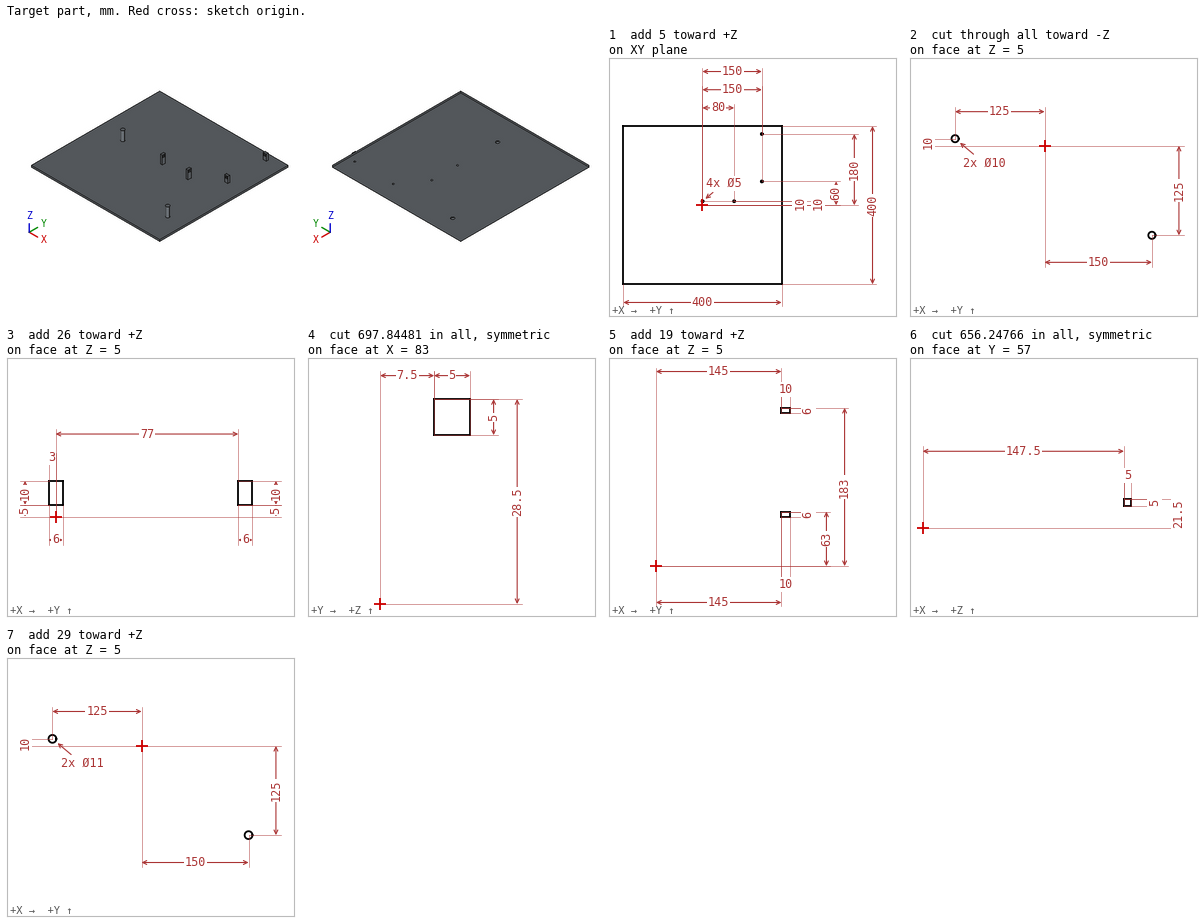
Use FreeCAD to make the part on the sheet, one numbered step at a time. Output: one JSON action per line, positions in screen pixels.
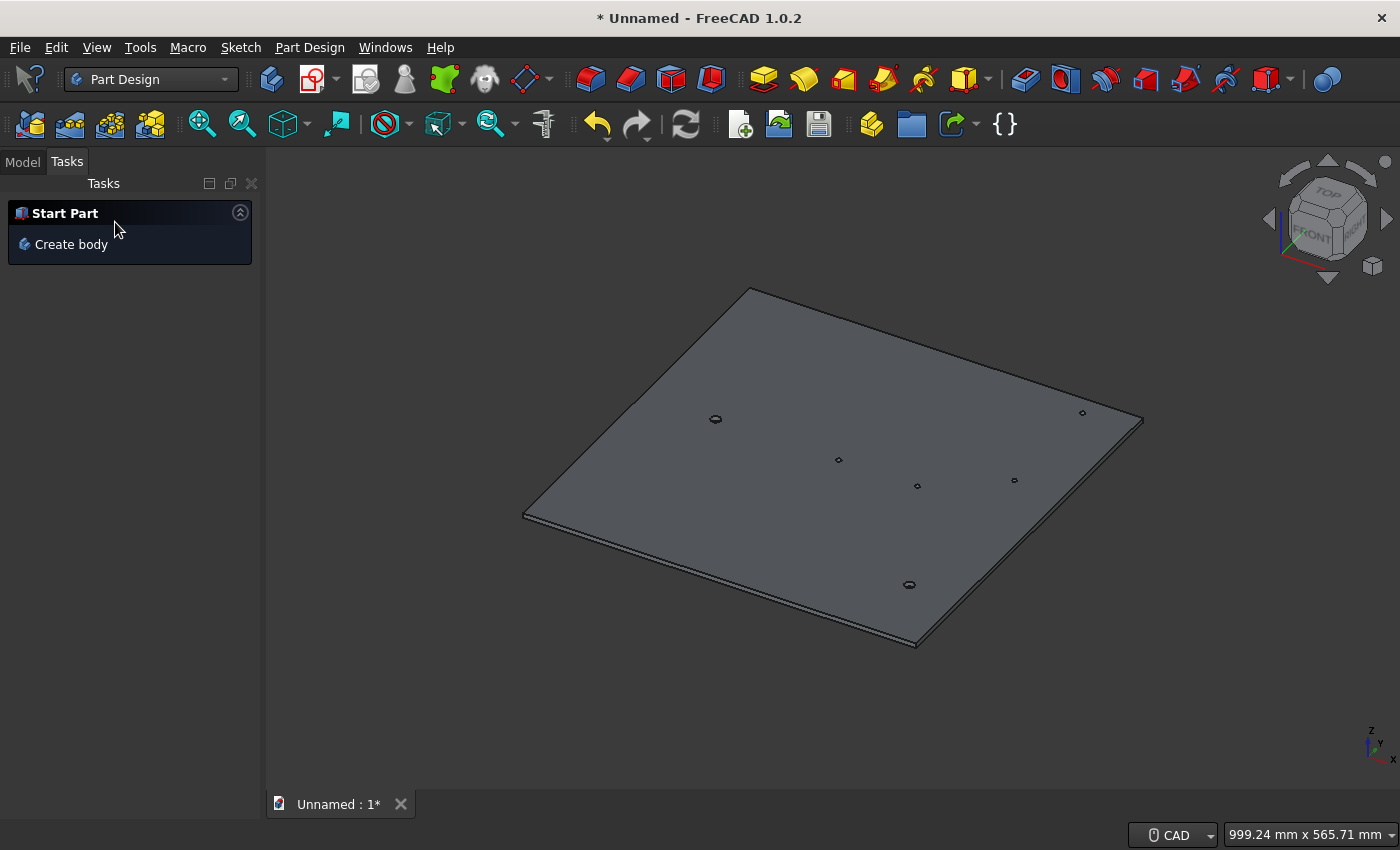
{"action": "left_click", "coordinate": [954, 419]}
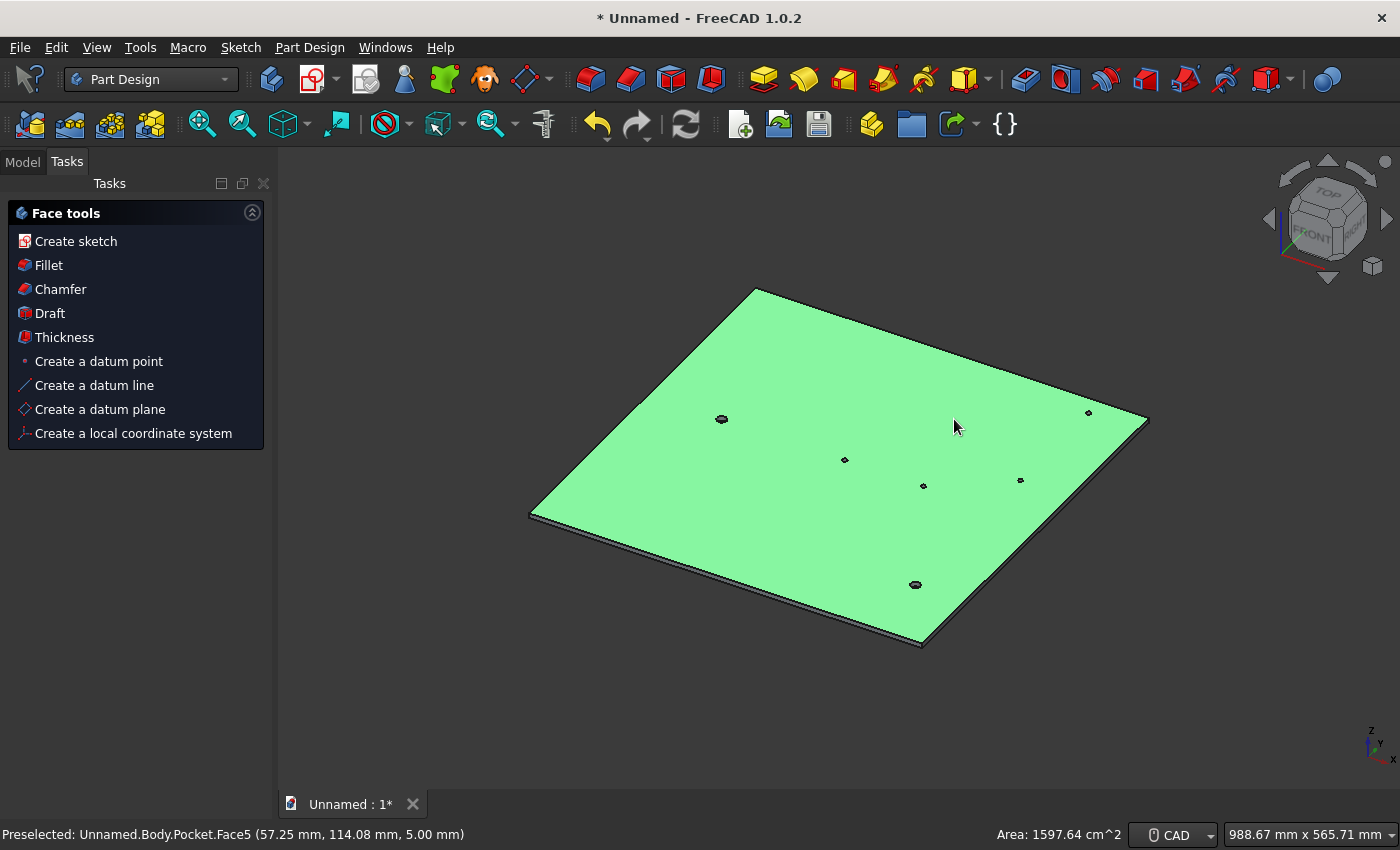
{"action": "left_click", "coordinate": [312, 80]}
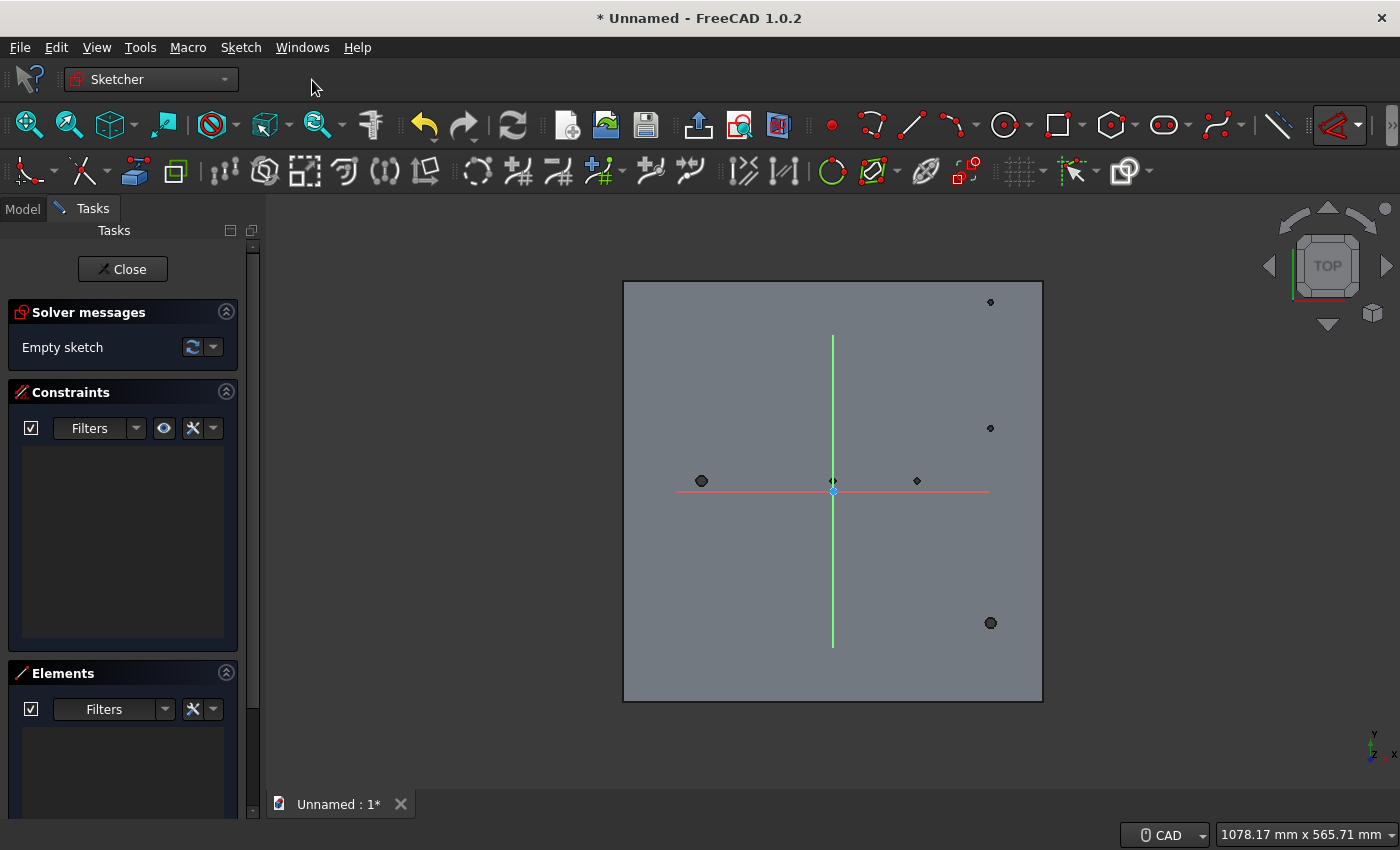
{"action": "scroll", "coordinate": [892, 482], "scroll_direction": "up", "scroll_amount": 10}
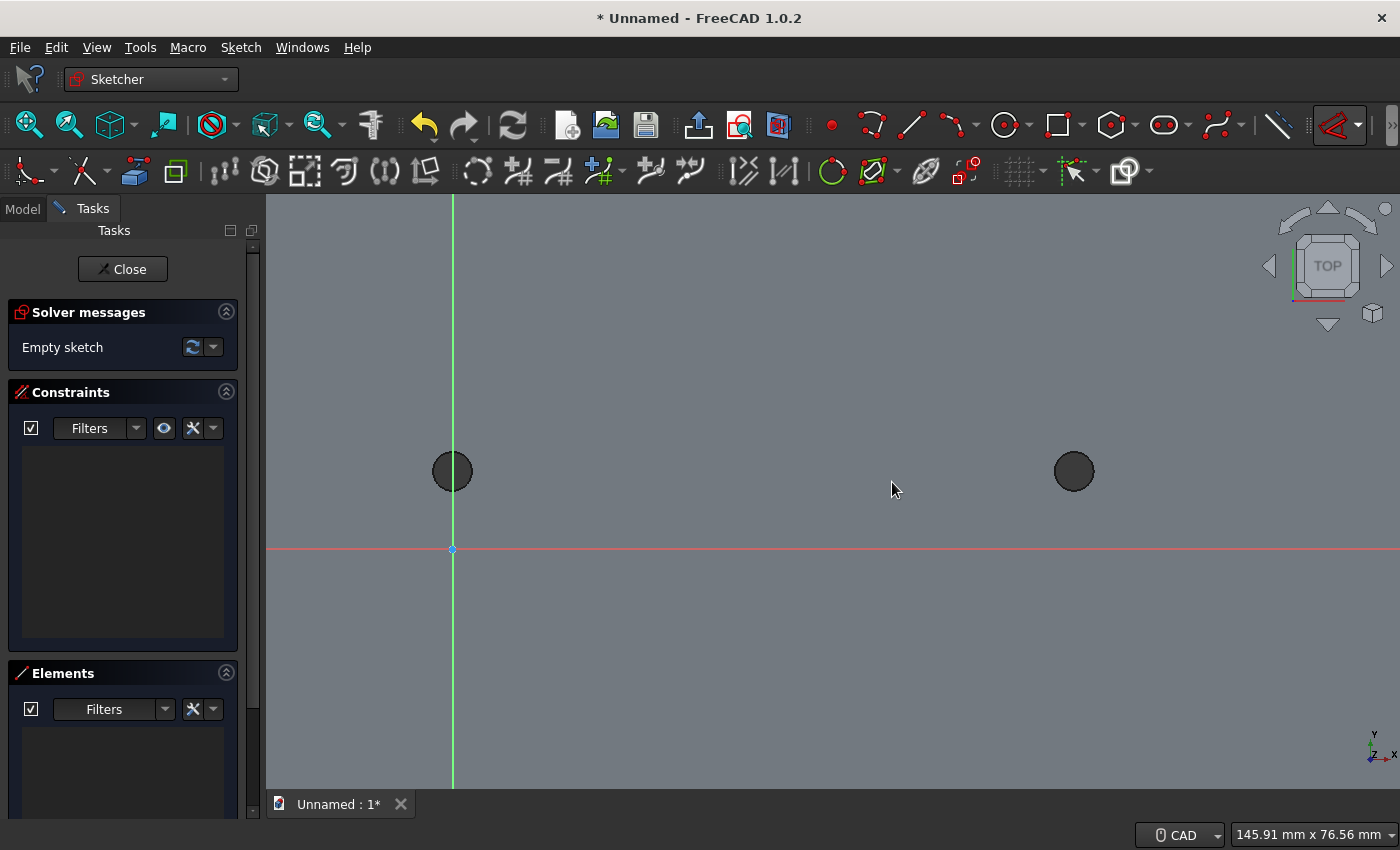
{"action": "key", "text": "g r"}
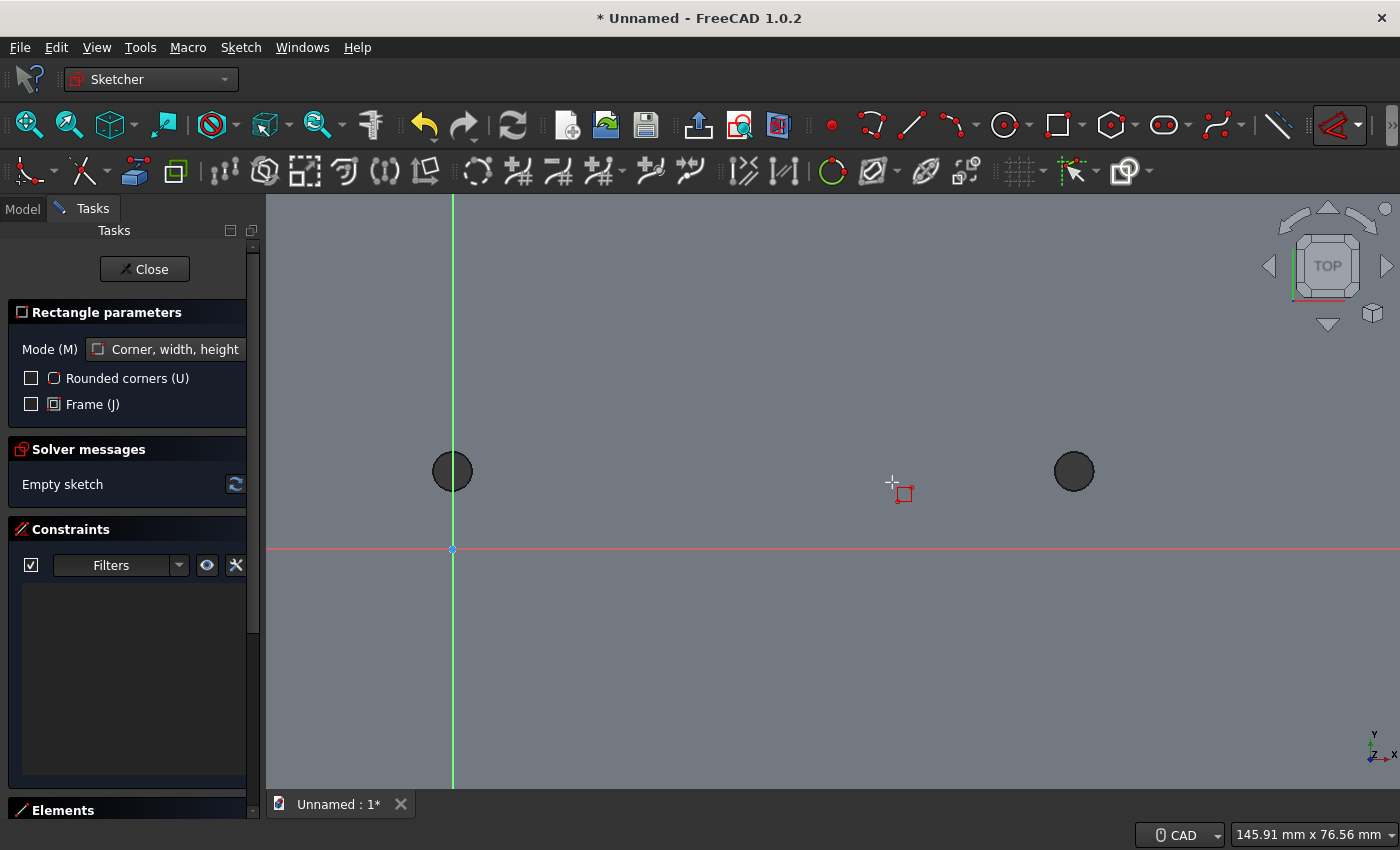
{"action": "left_click", "coordinate": [429, 433]}
{"action": "left_click", "coordinate": [476, 510]}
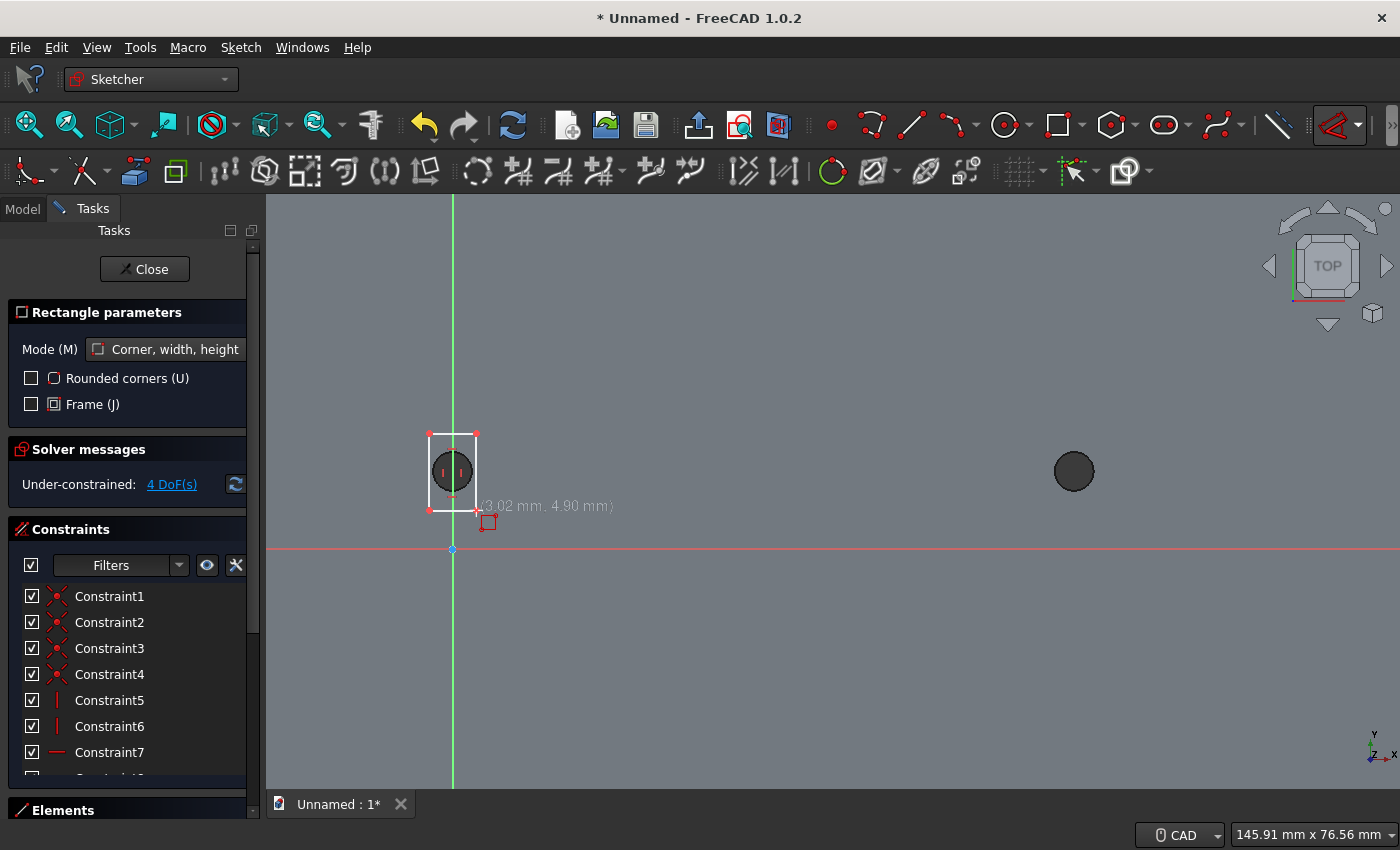
{"action": "left_click", "coordinate": [1051, 433]}
{"action": "left_click", "coordinate": [1098, 510]}
{"action": "key", "text": "Escape"}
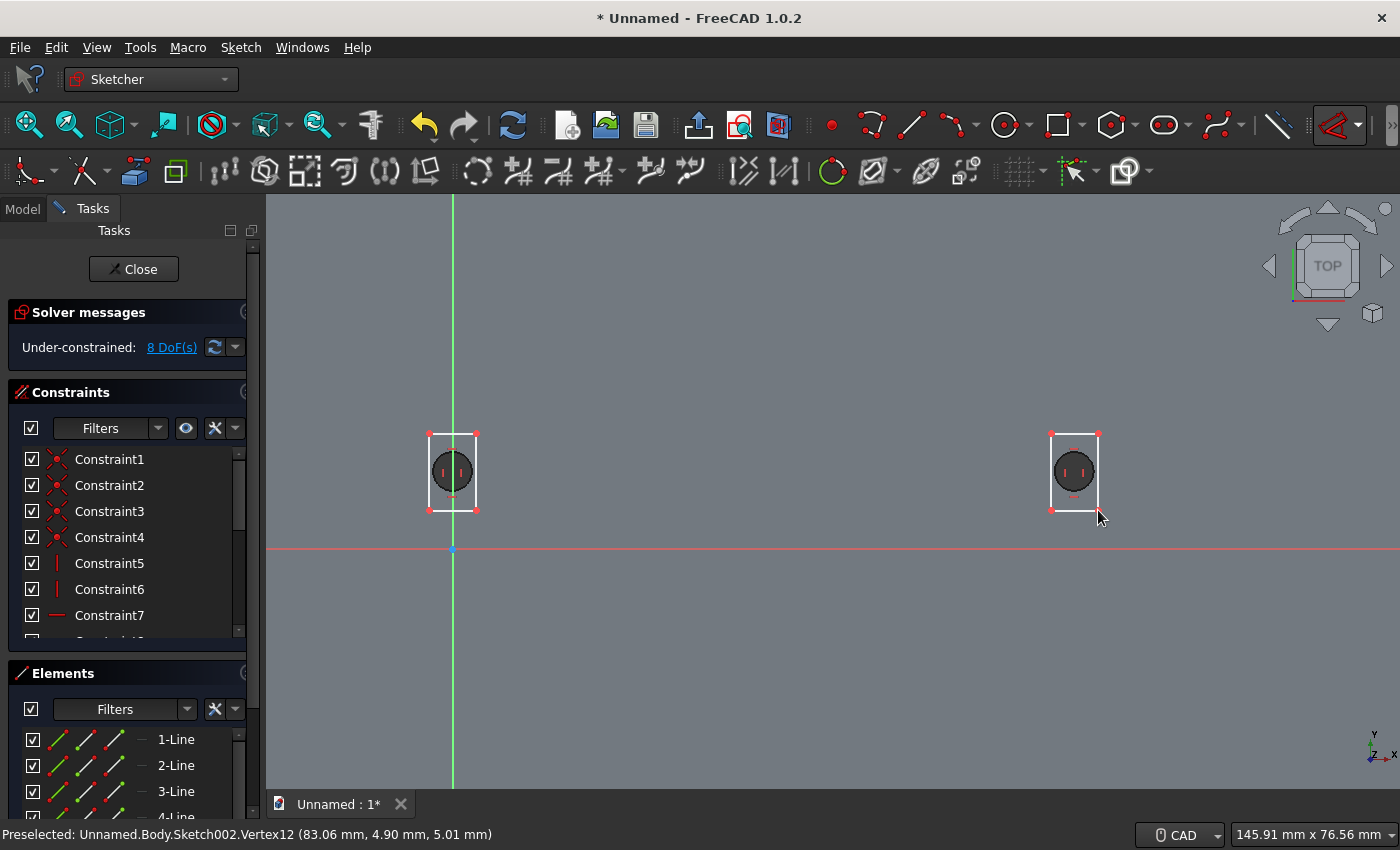
{"action": "scroll", "coordinate": [443, 511], "scroll_direction": "up", "scroll_amount": 2}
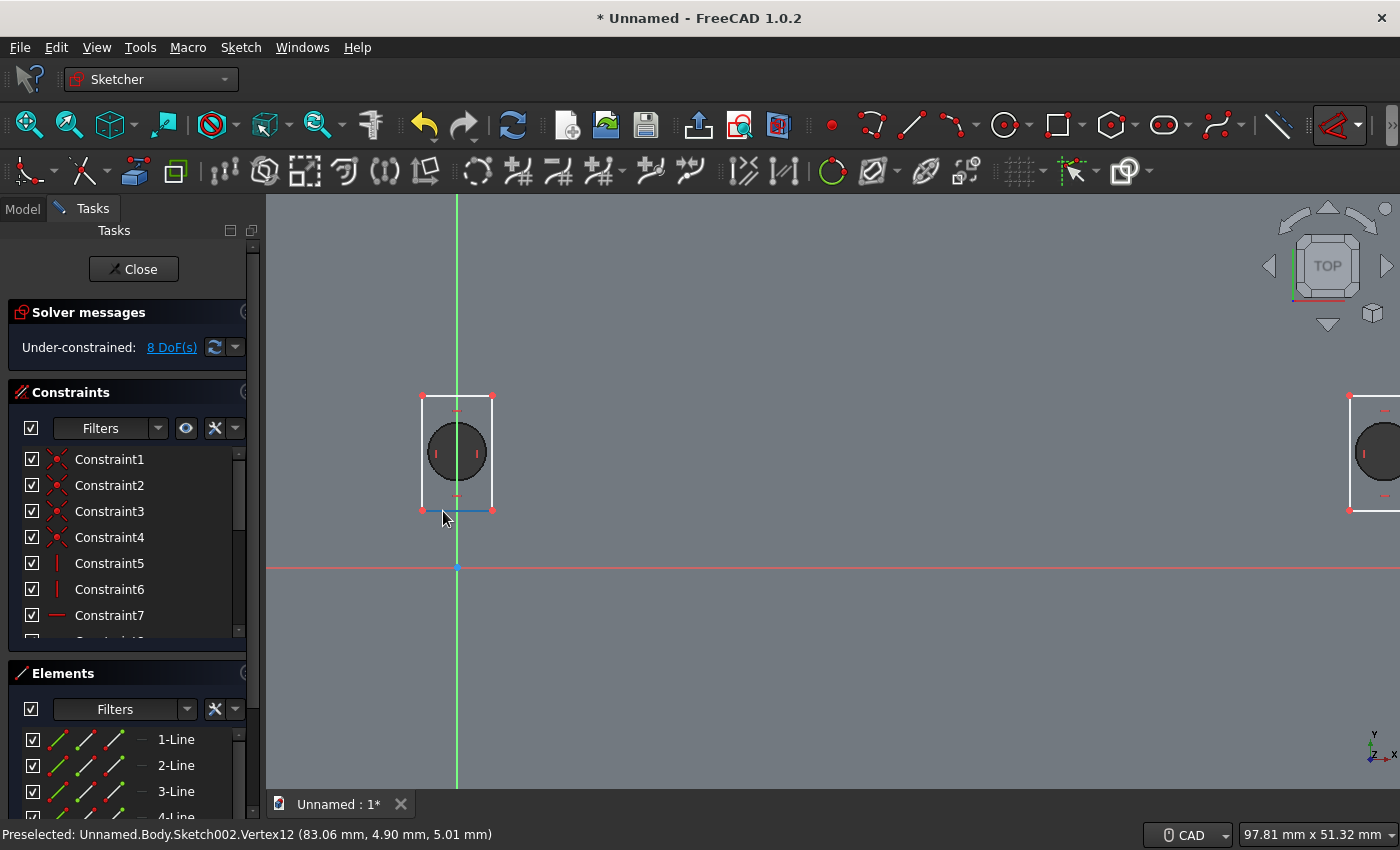
{"action": "left_click", "coordinate": [443, 511]}